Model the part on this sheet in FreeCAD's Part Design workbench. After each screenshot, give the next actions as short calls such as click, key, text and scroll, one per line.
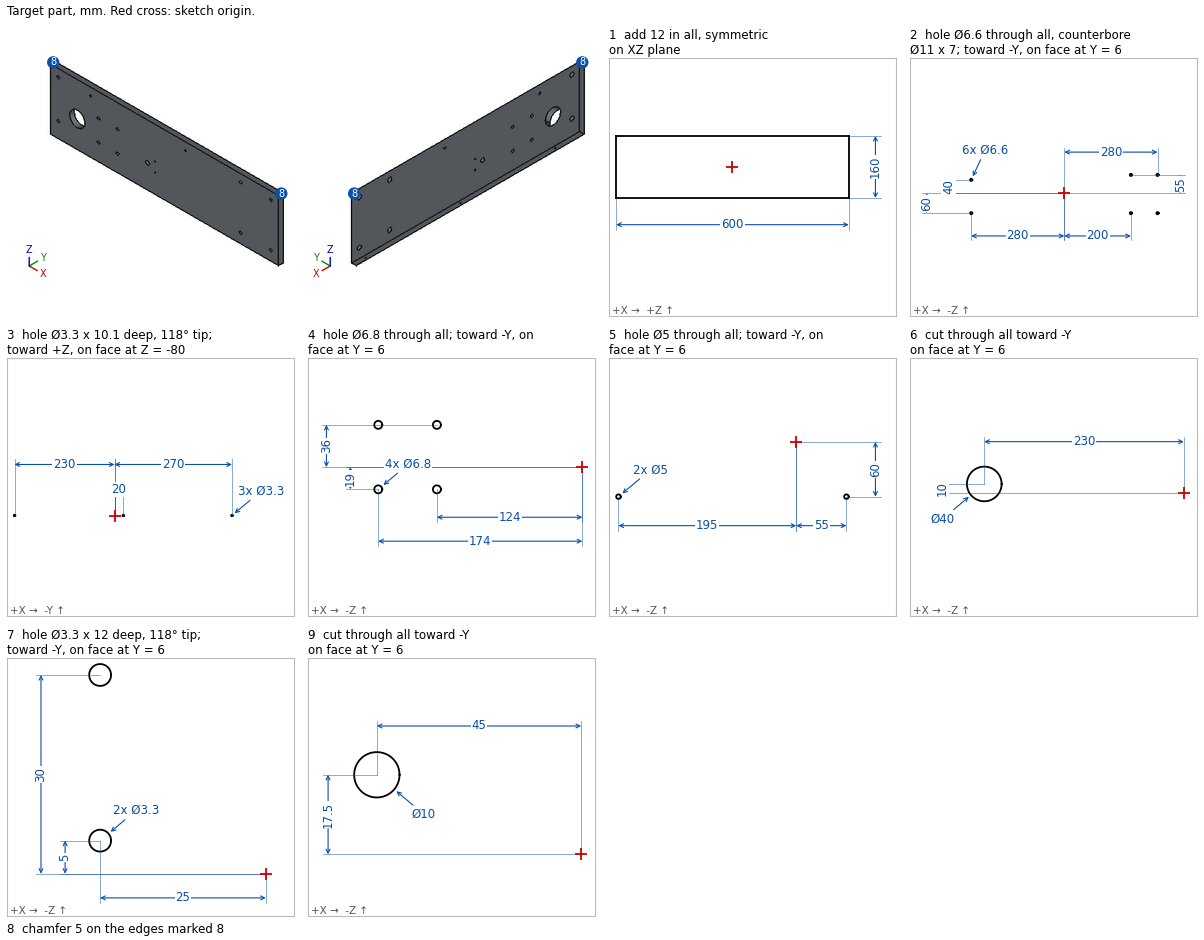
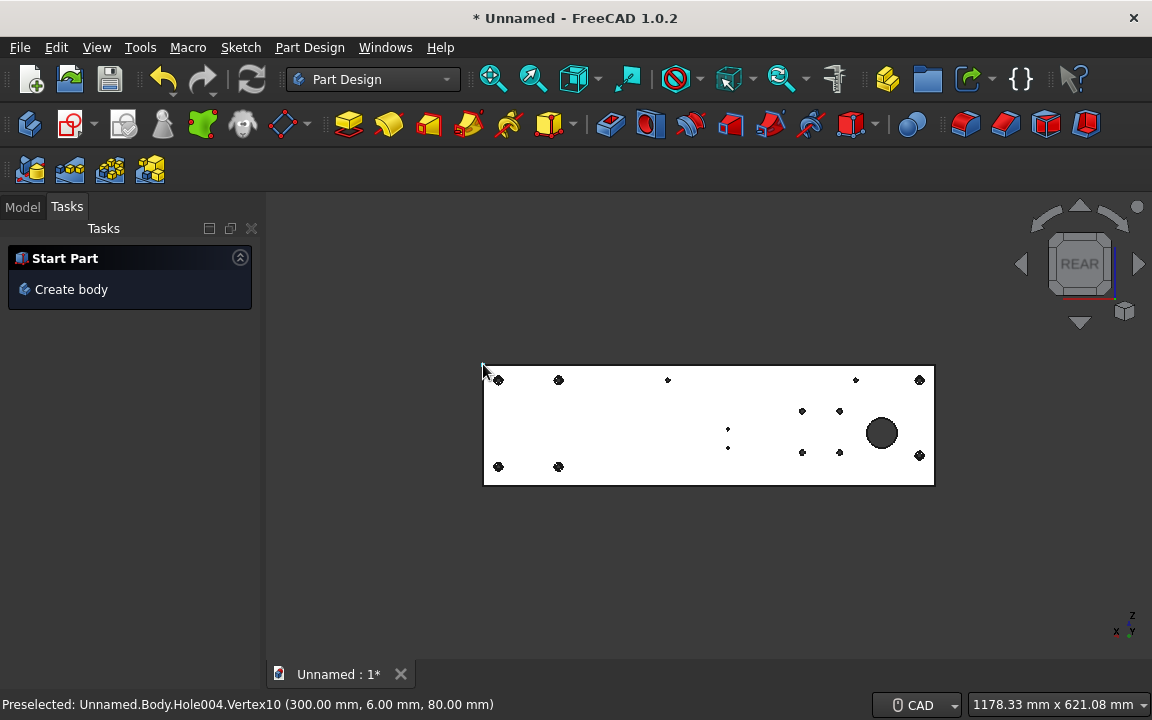
key(0)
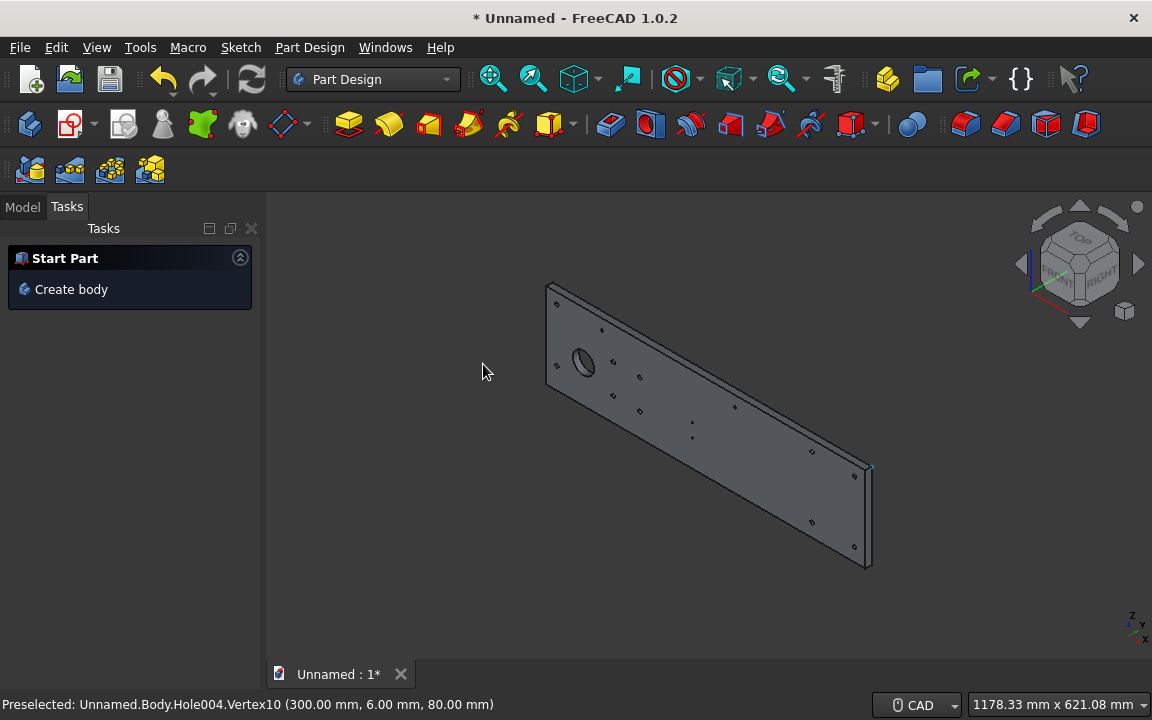
scroll(869, 467, up, 8)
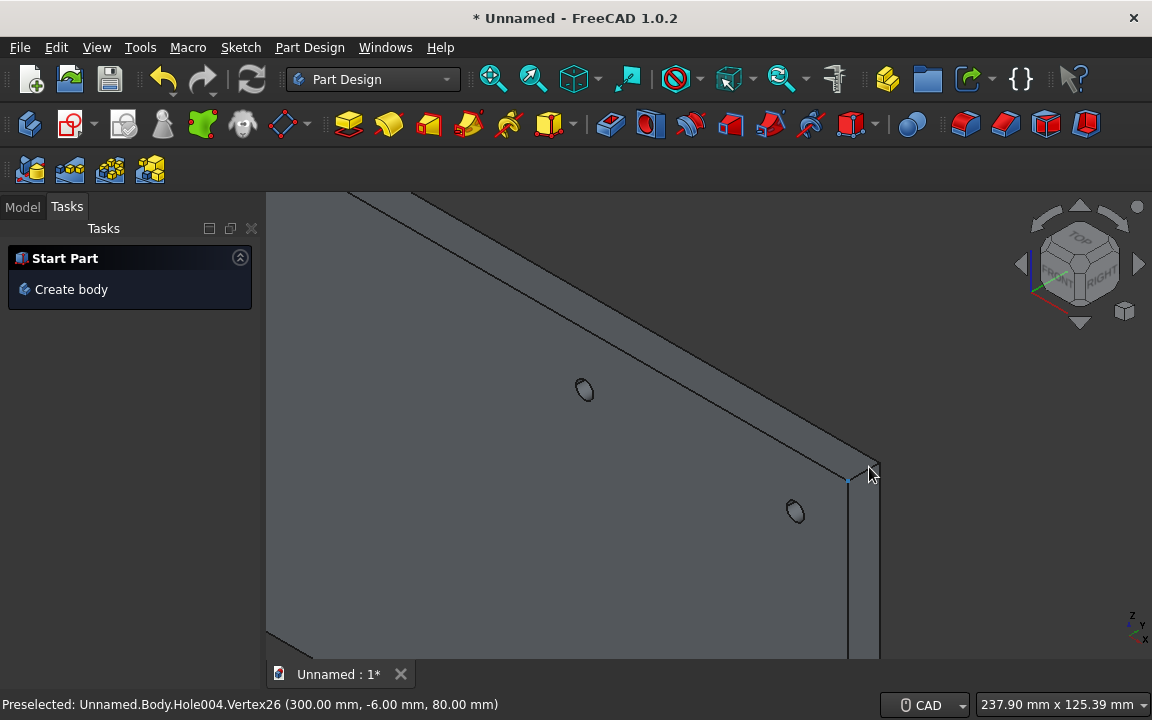
click(864, 471)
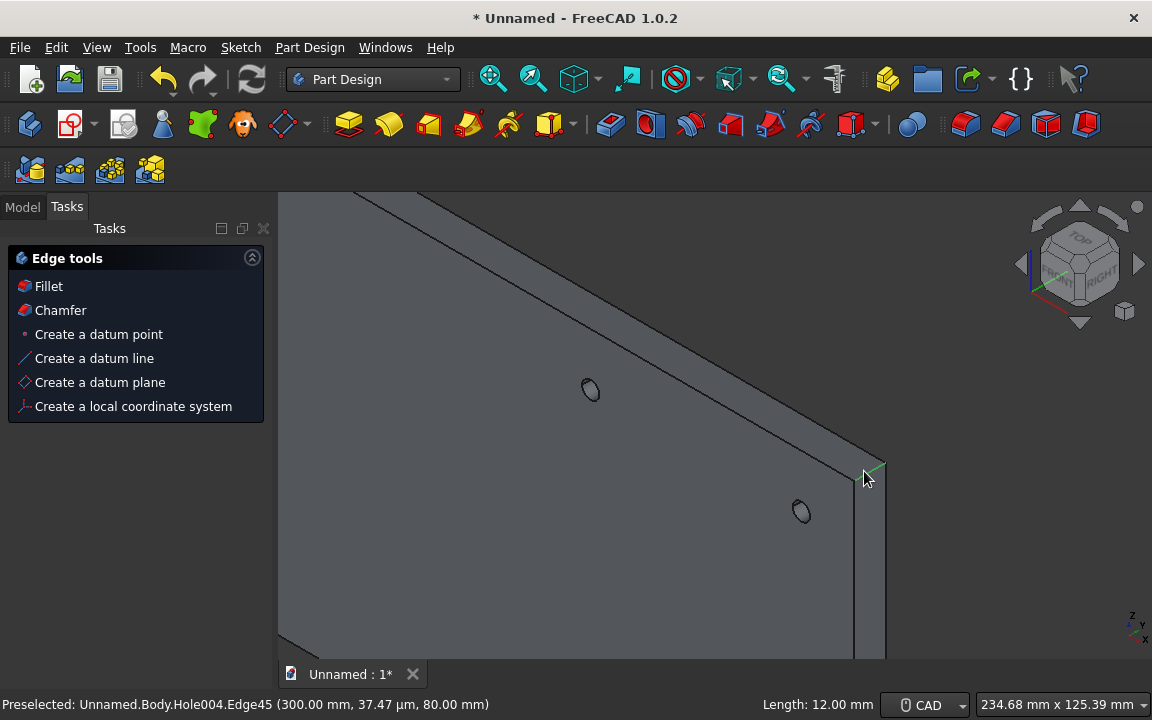
click(494, 80)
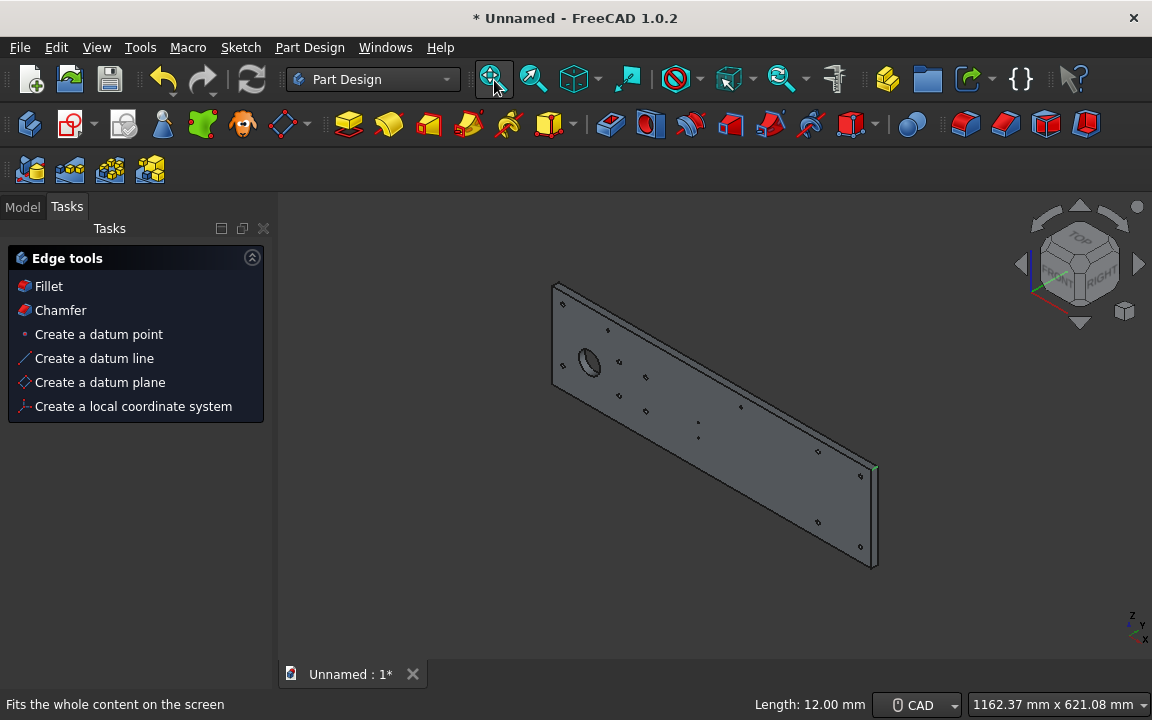
key(2)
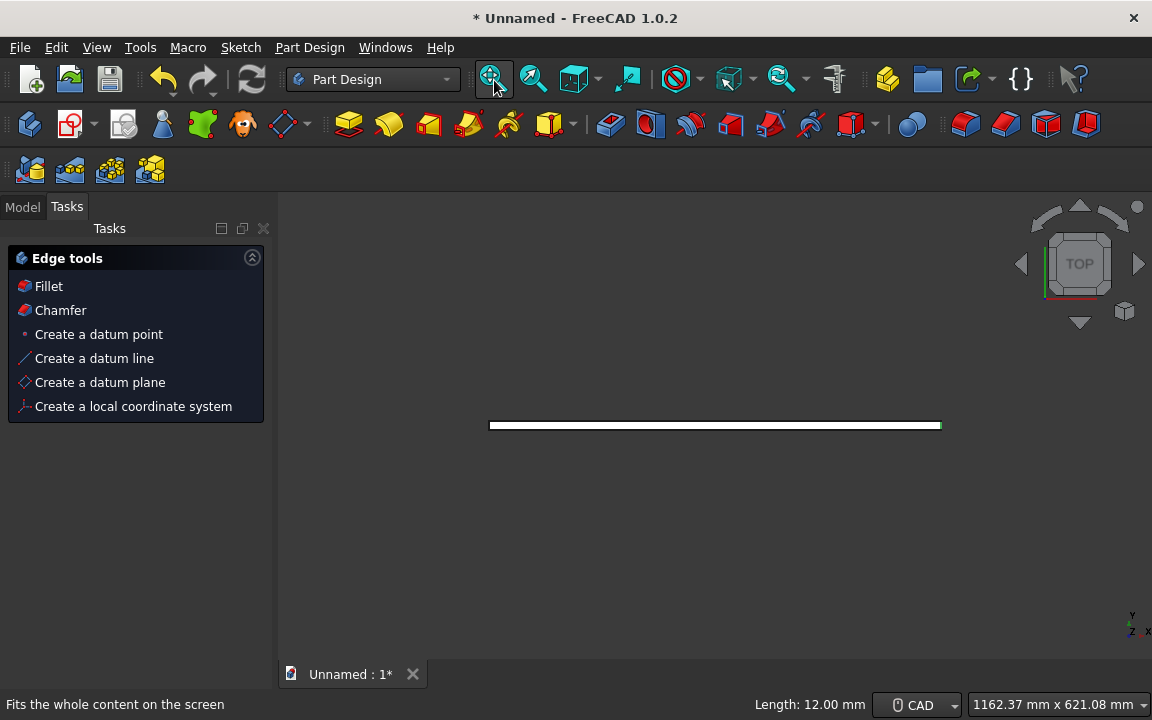
click(489, 426, ctrl)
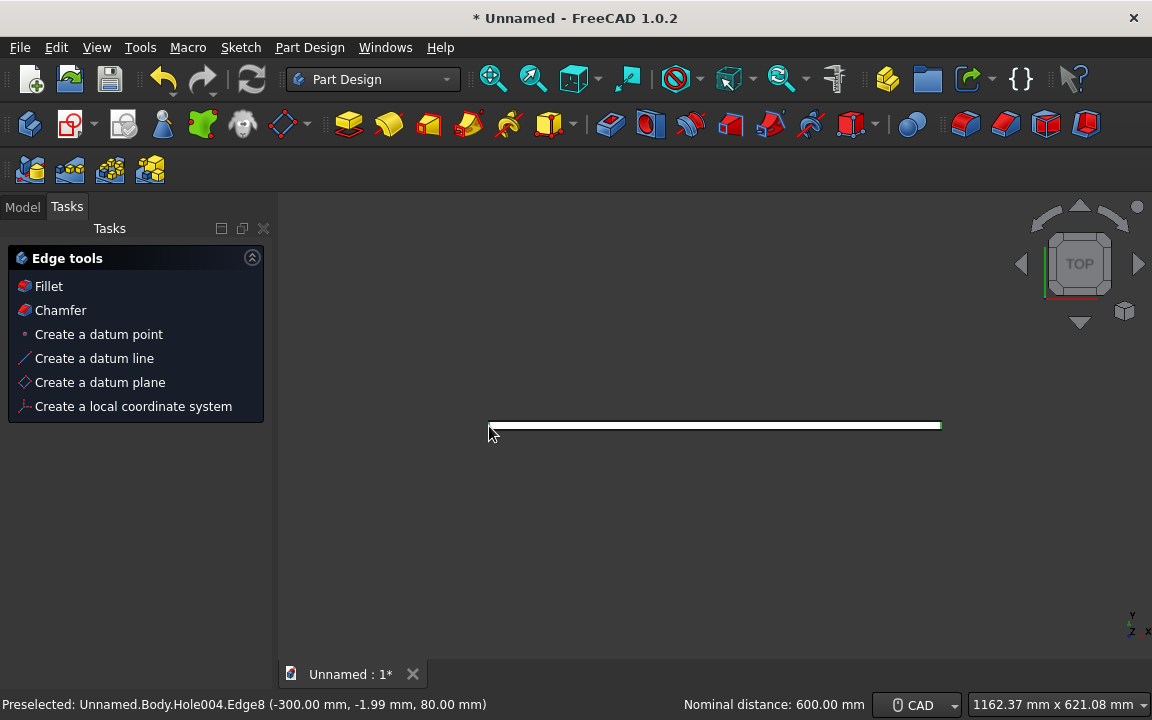
click(1006, 124)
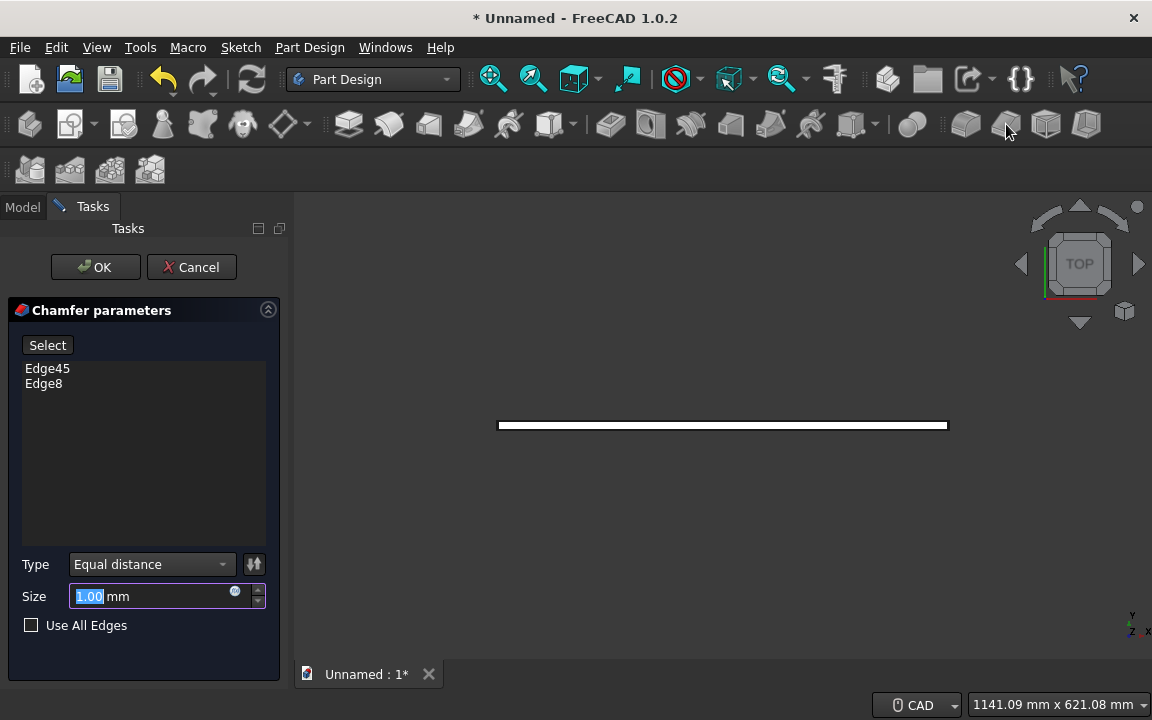
text(5)
key(Tab)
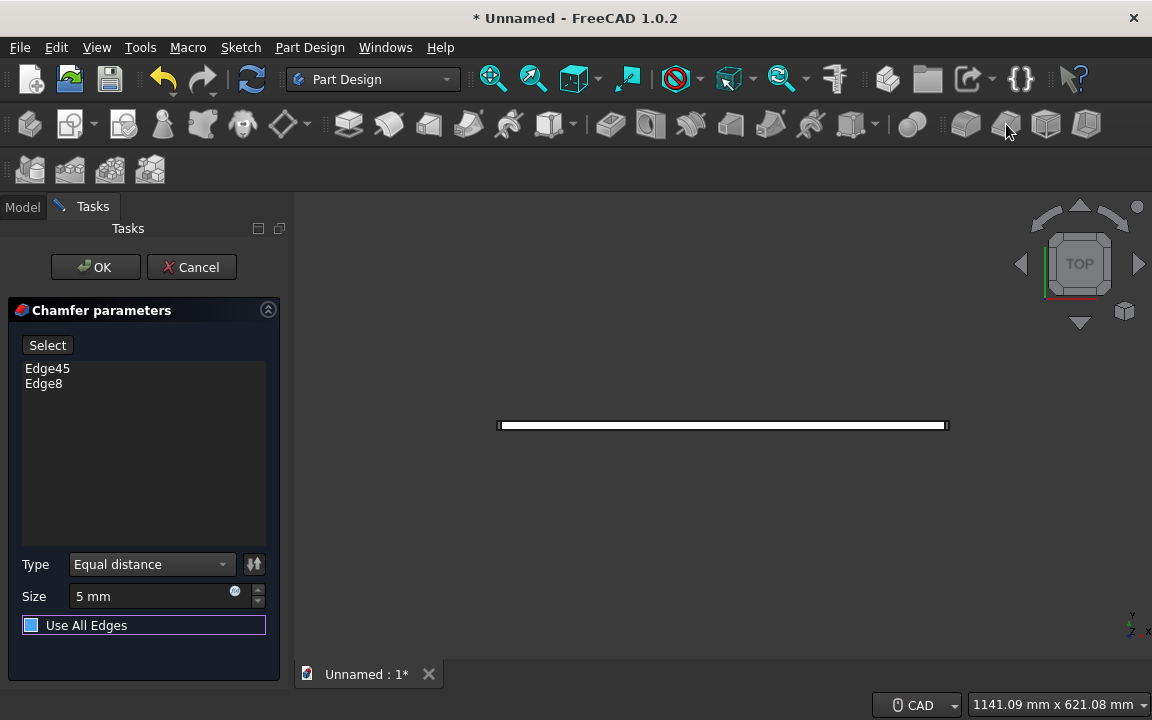
click(96, 267)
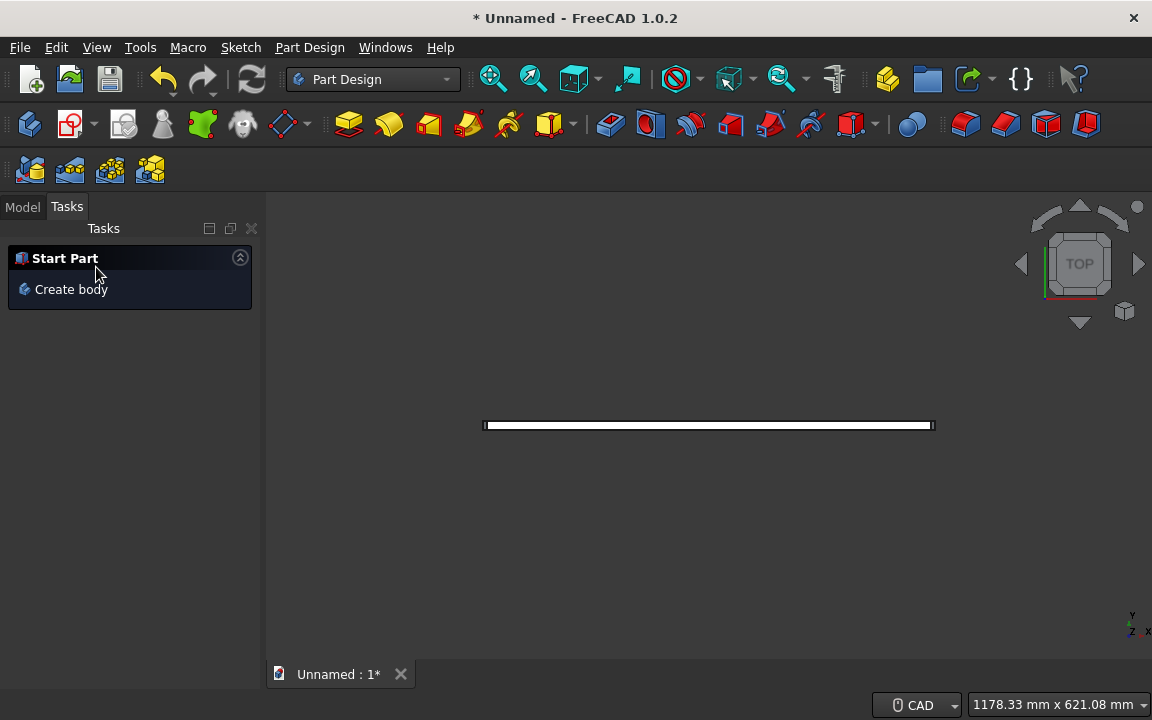
key(4)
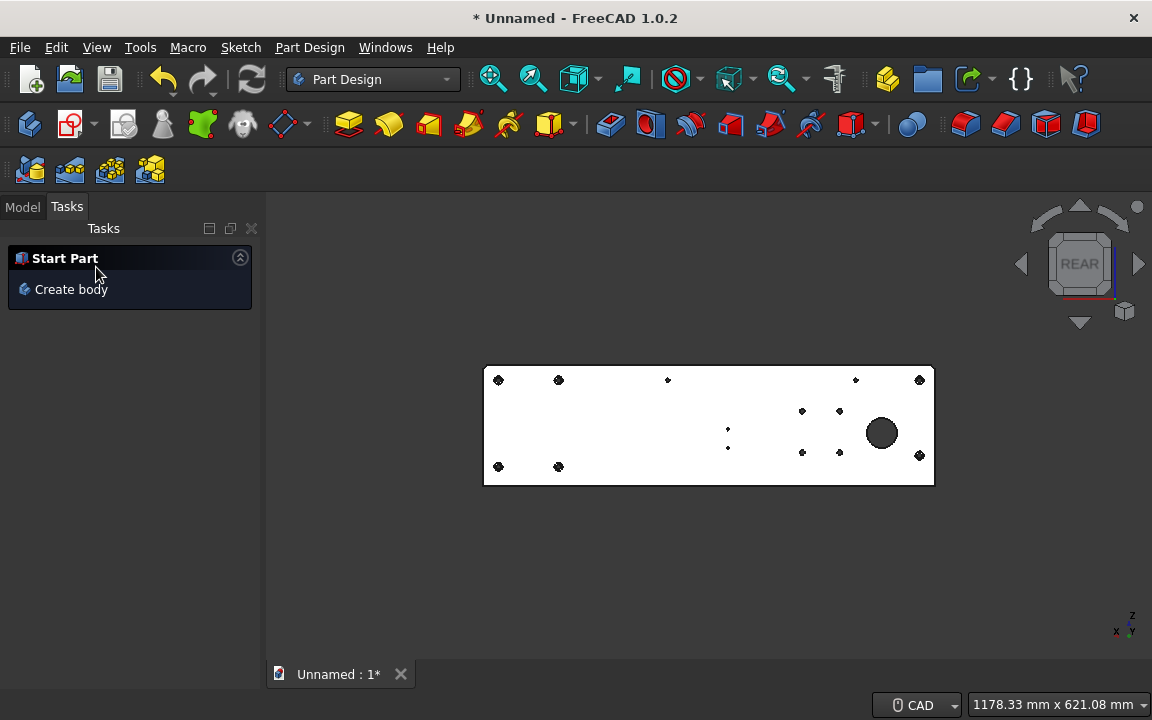
click(645, 424)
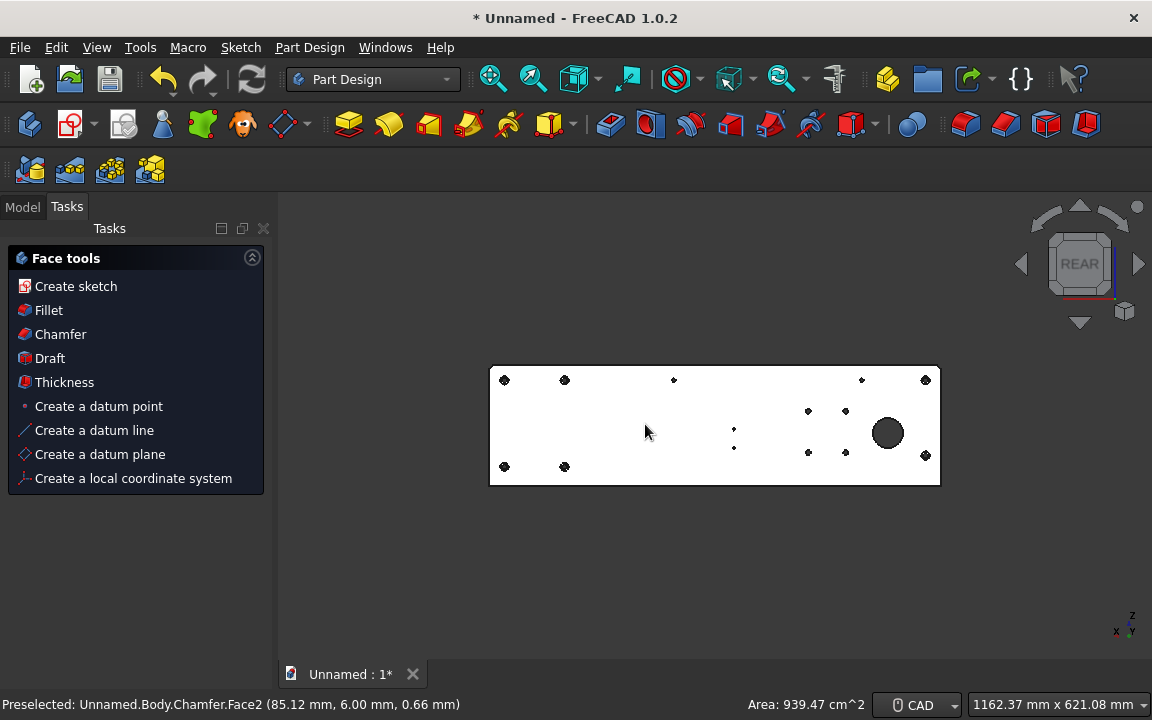
click(70, 124)